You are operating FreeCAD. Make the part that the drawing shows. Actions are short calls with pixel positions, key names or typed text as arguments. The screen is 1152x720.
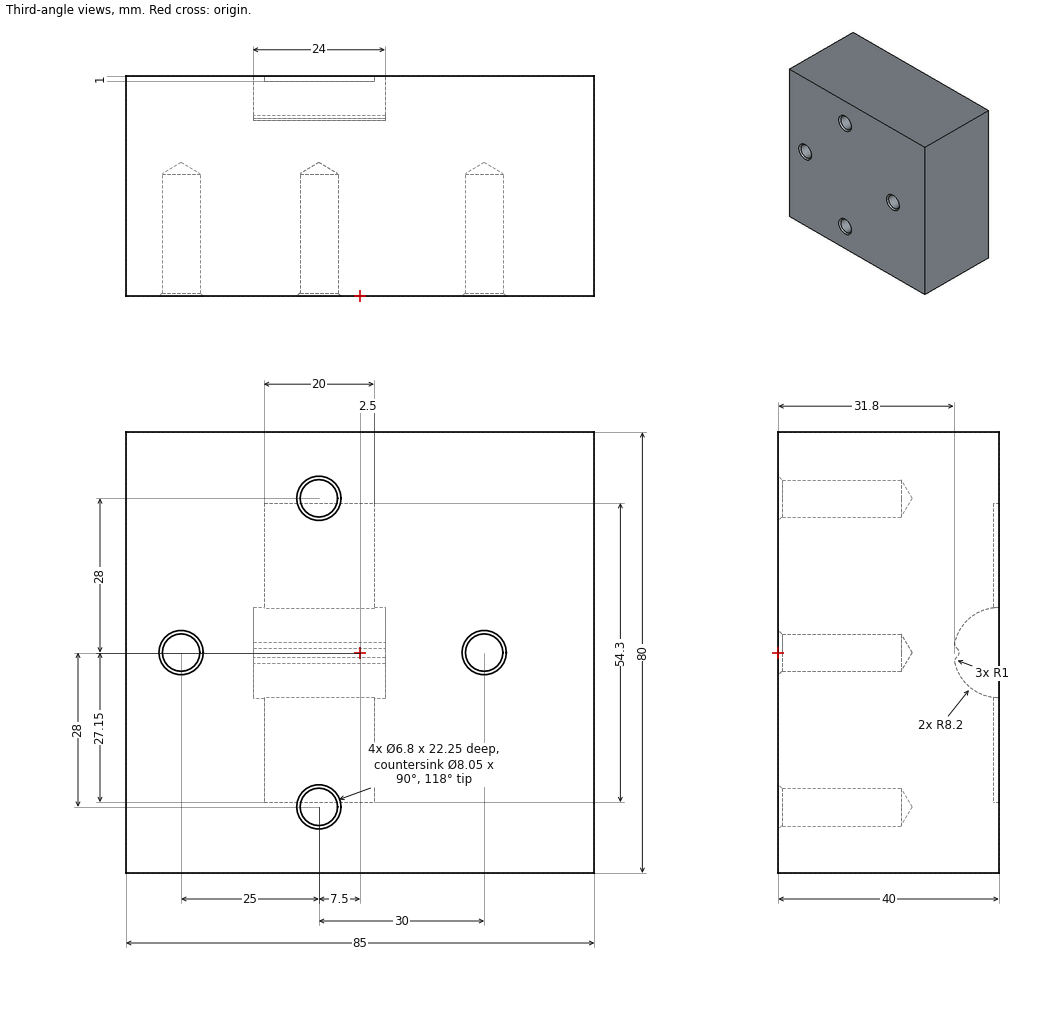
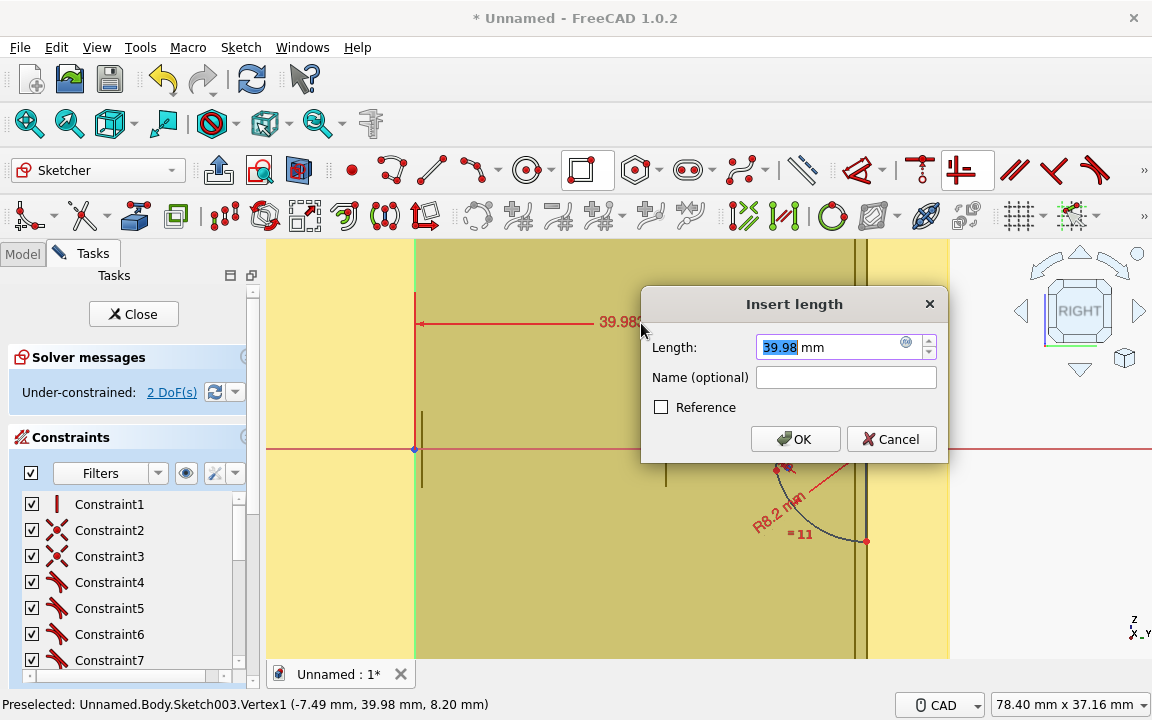
text(40)
key(Return)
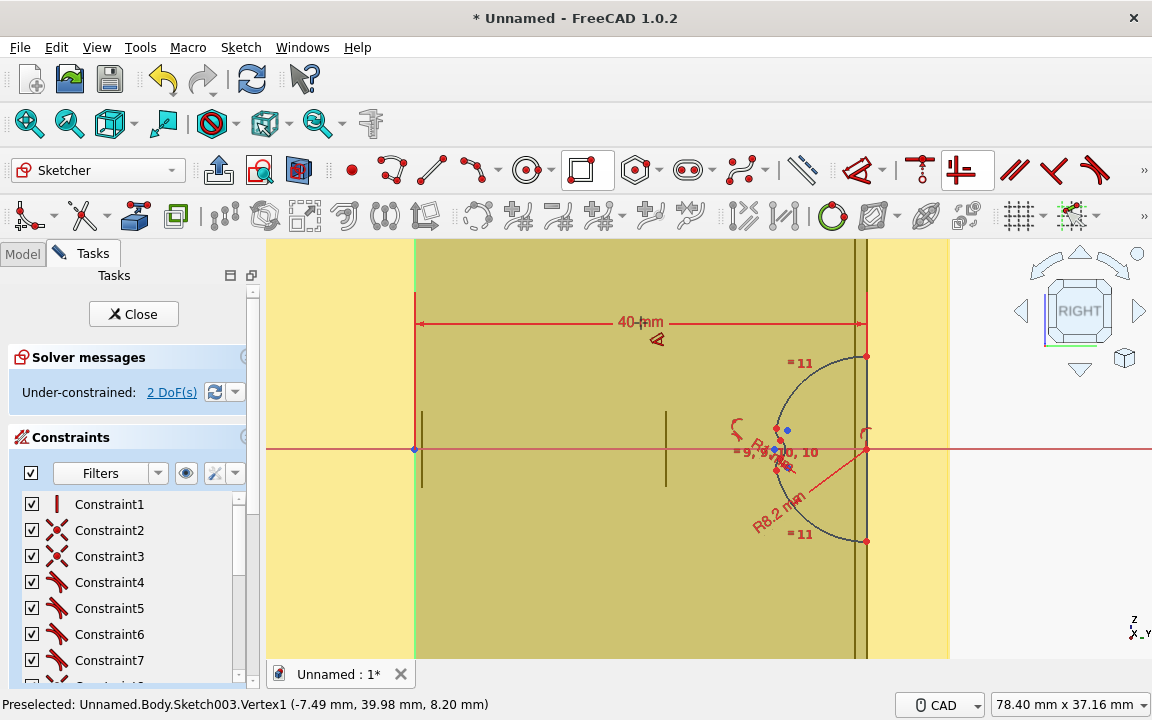
click(867, 449)
click(641, 483)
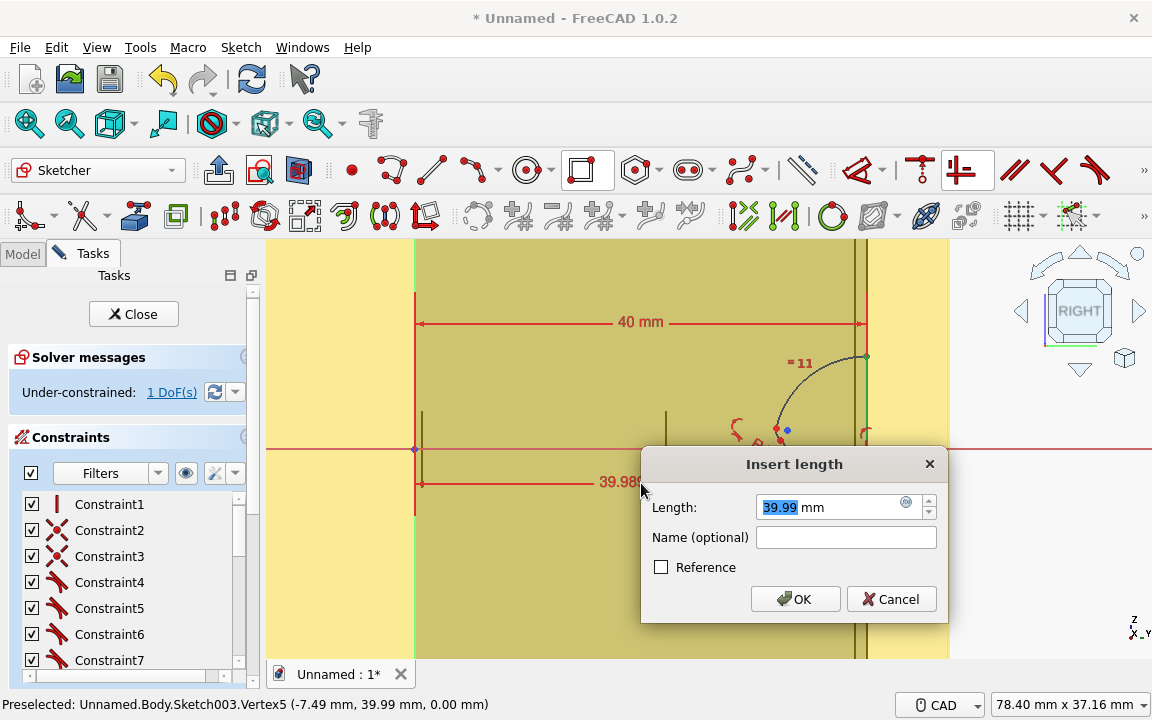
text(40)
key(Return)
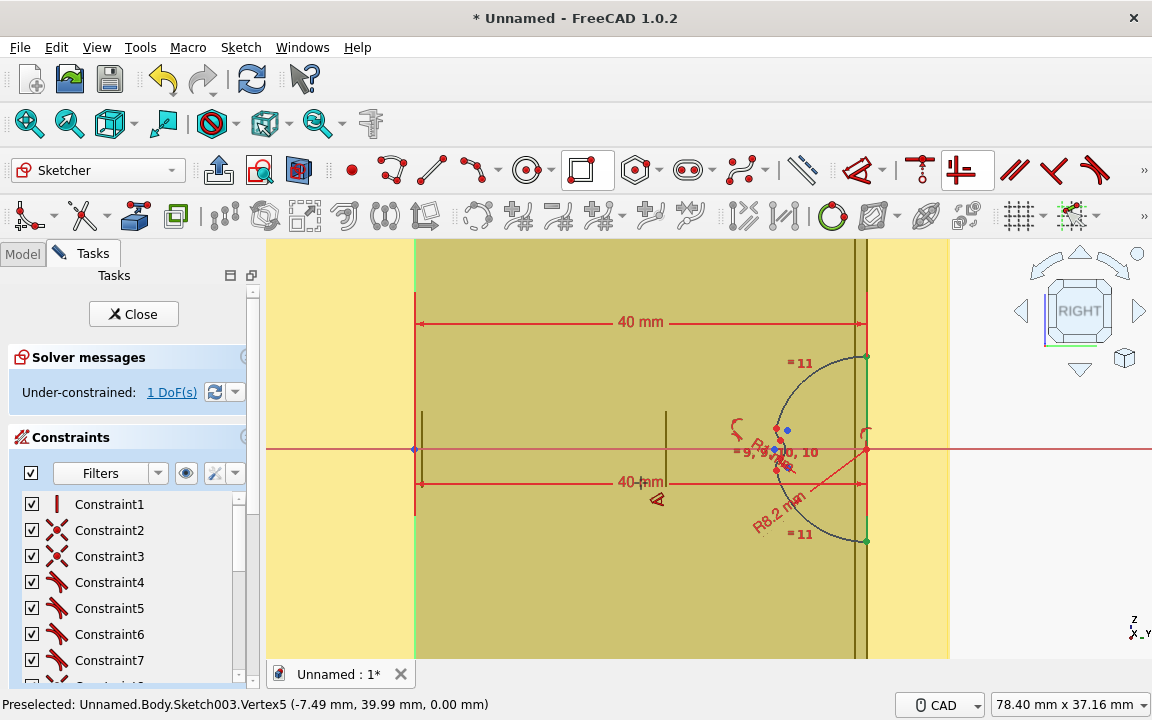
click(774, 449)
click(512, 483)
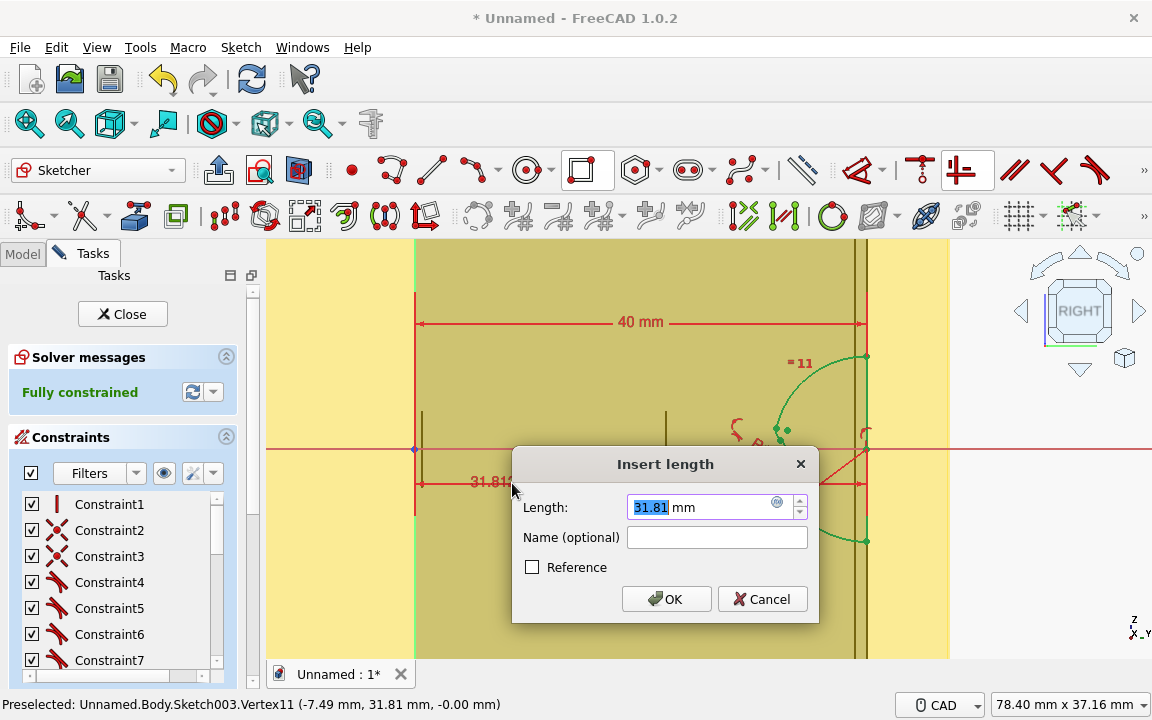
text(31.8)
key(Return)
key(Escape)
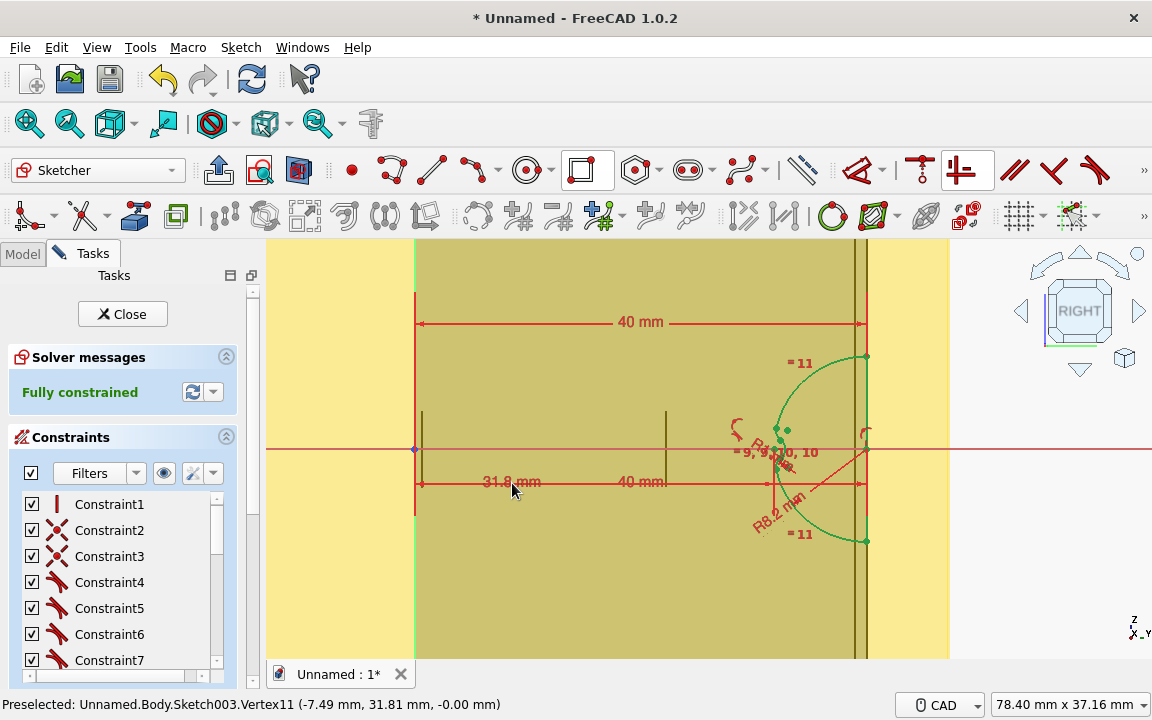
click(123, 314)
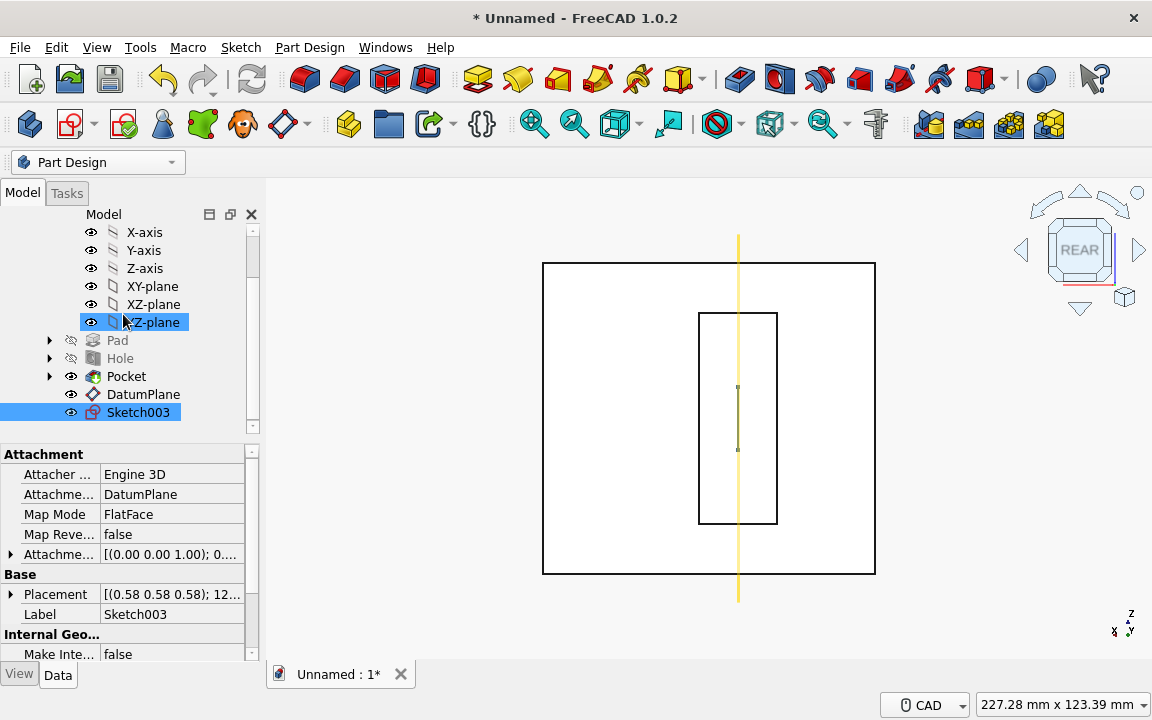
click(740, 80)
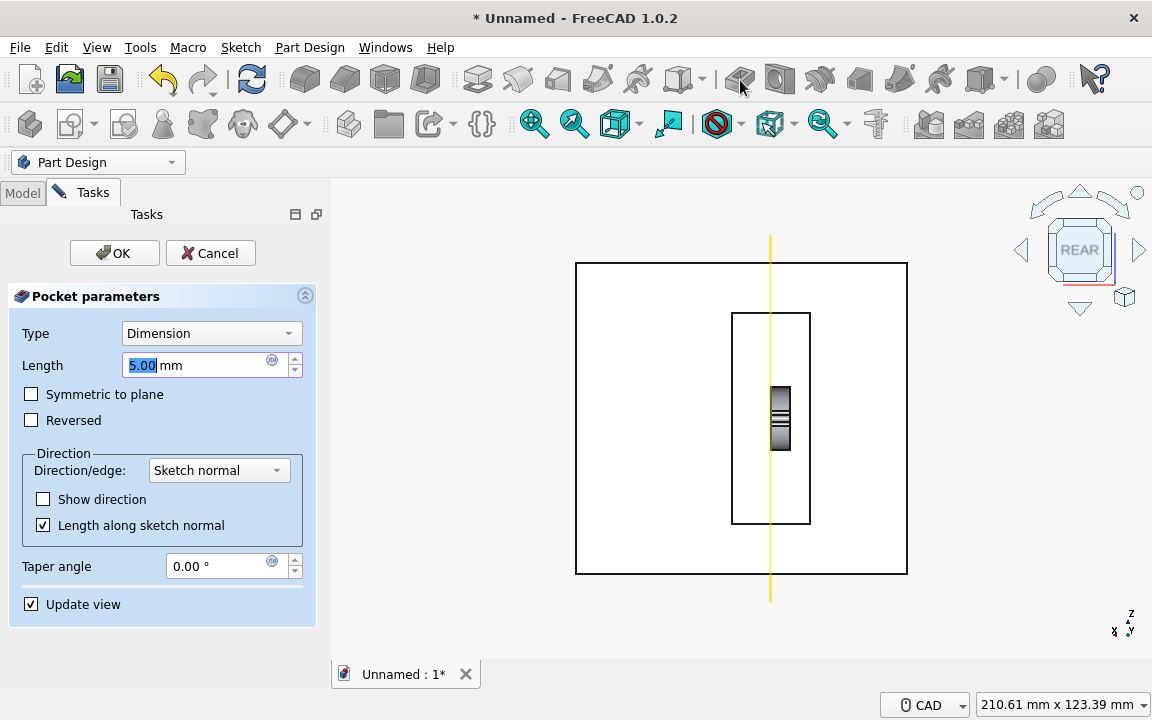
text(24)
key(Tab)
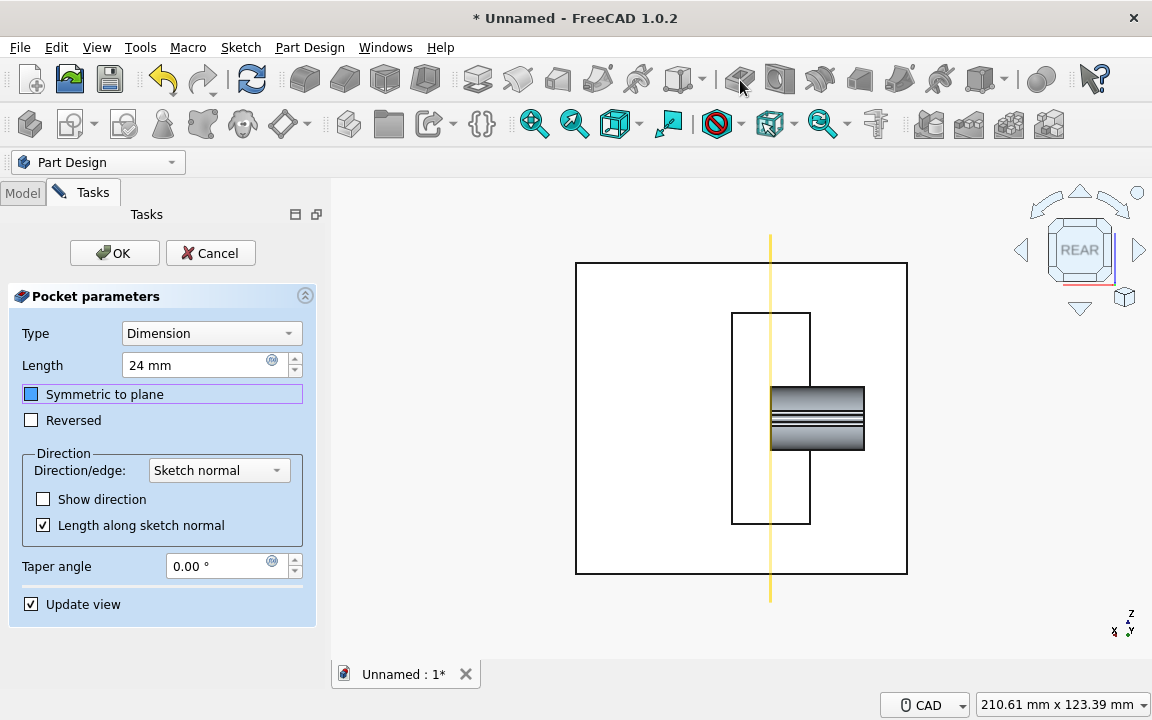
click(30, 394)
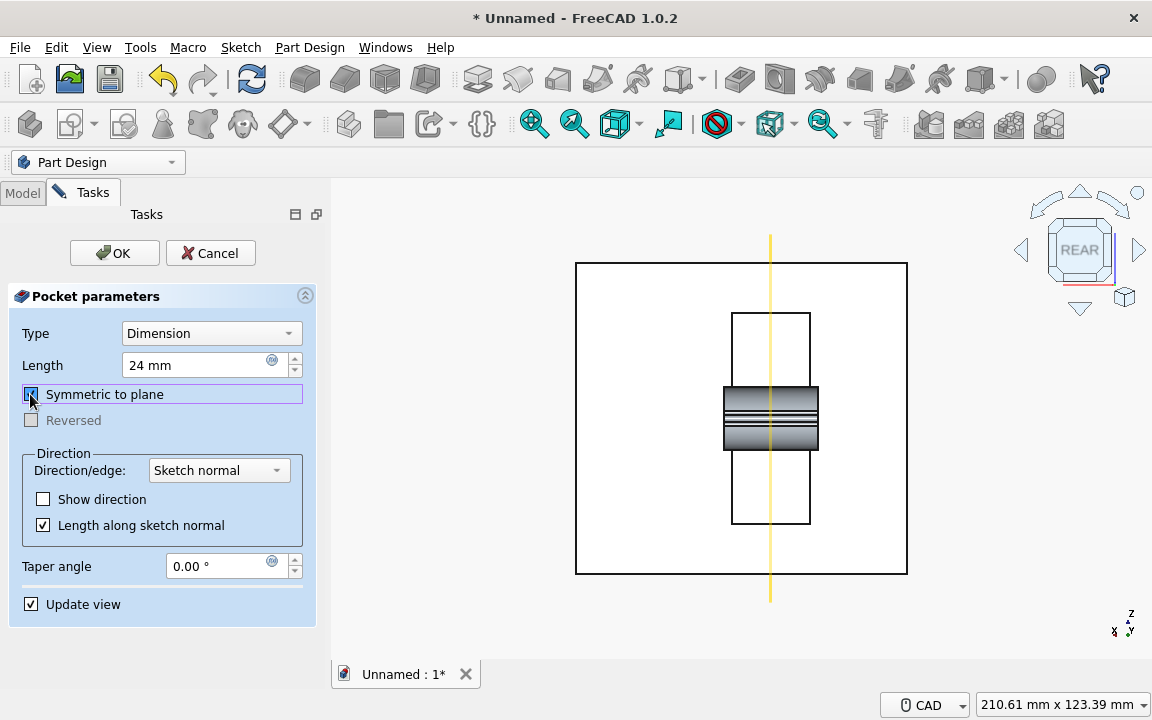
click(115, 253)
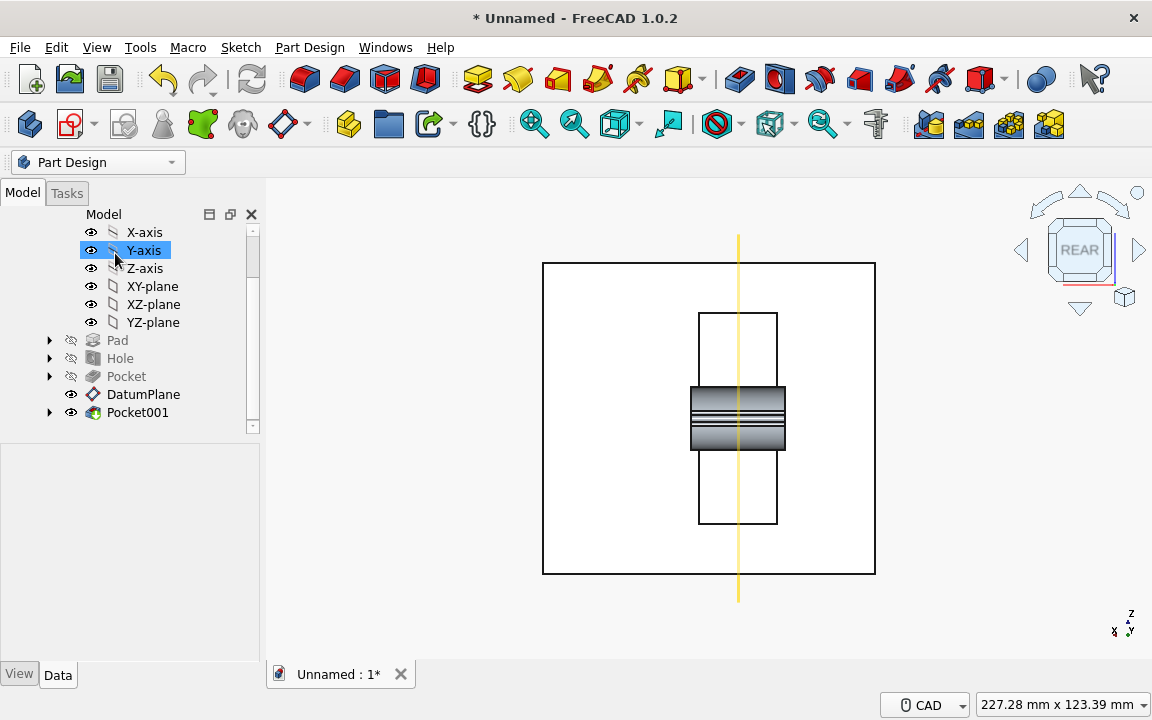
click(116, 394)
key(space)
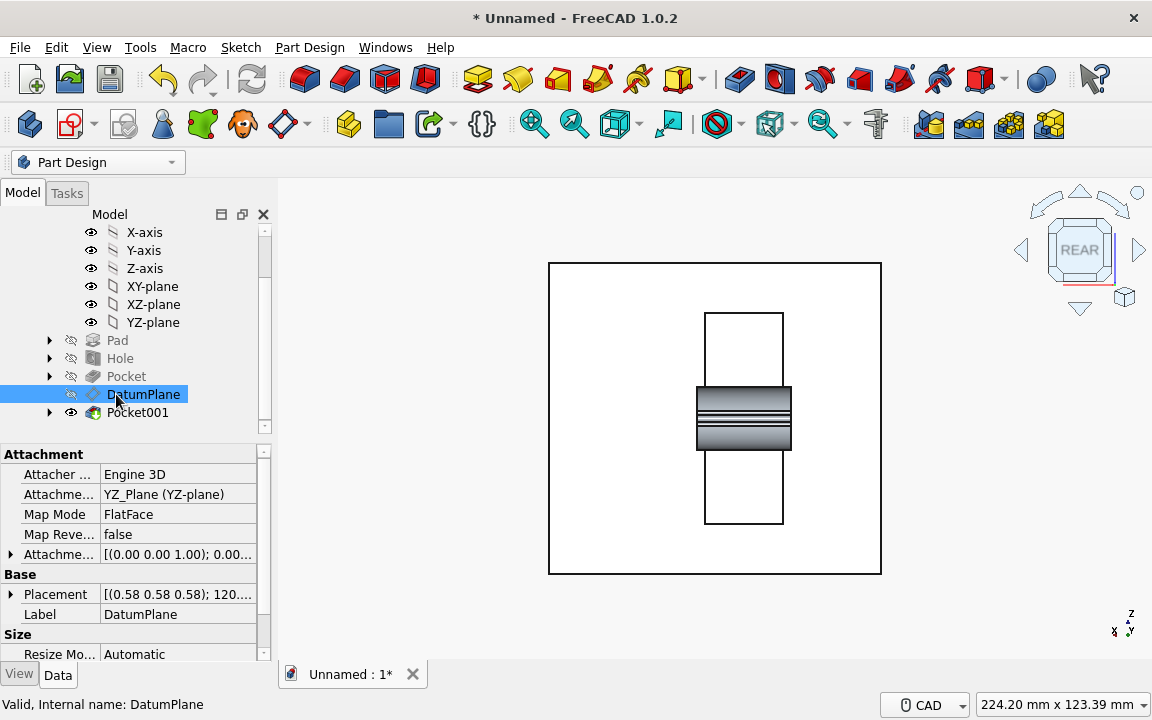
key(0)